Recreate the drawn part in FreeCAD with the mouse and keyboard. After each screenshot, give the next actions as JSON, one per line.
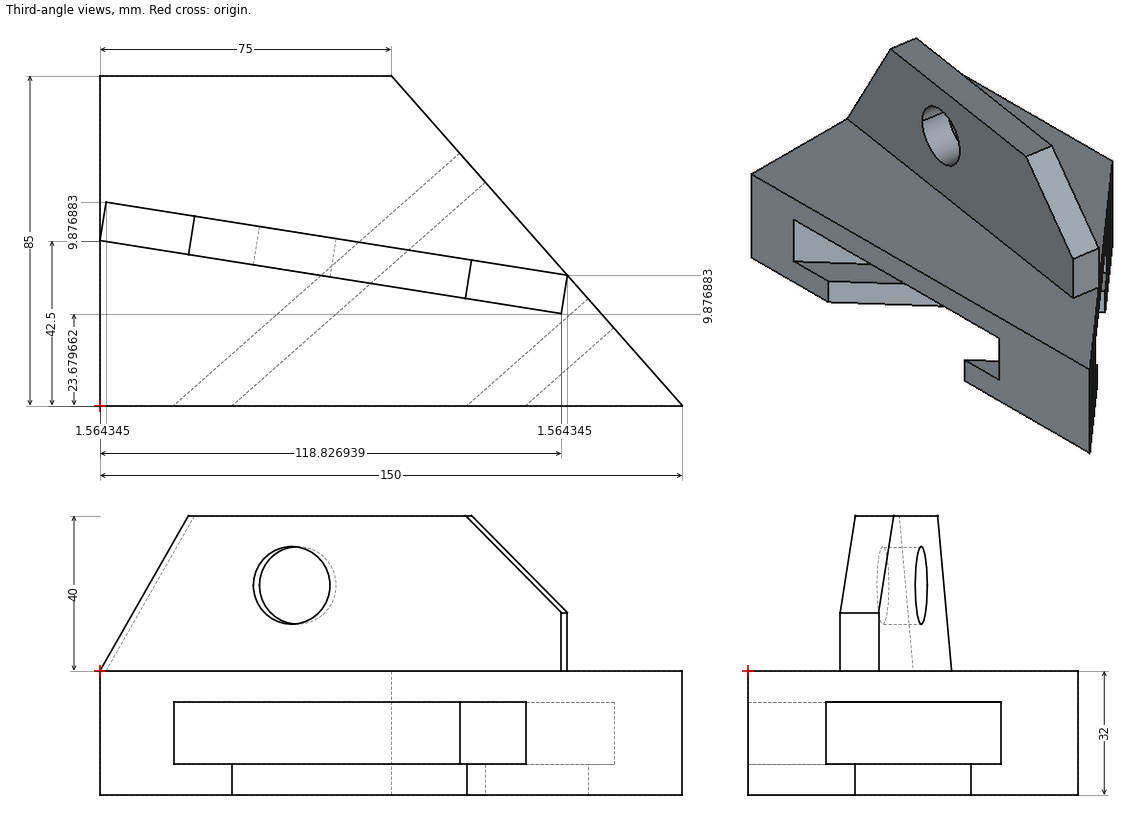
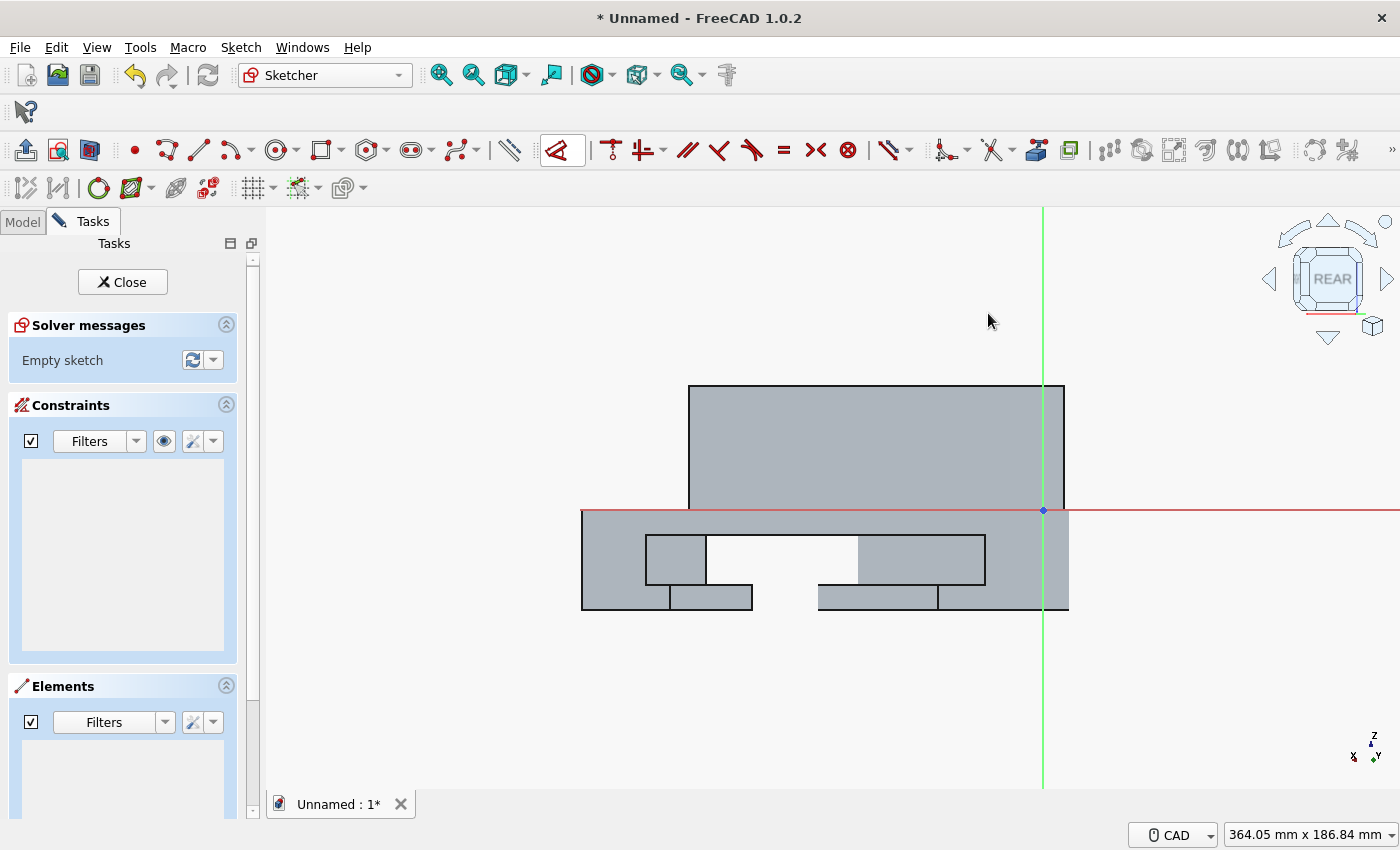
{"action": "key", "text": "g m"}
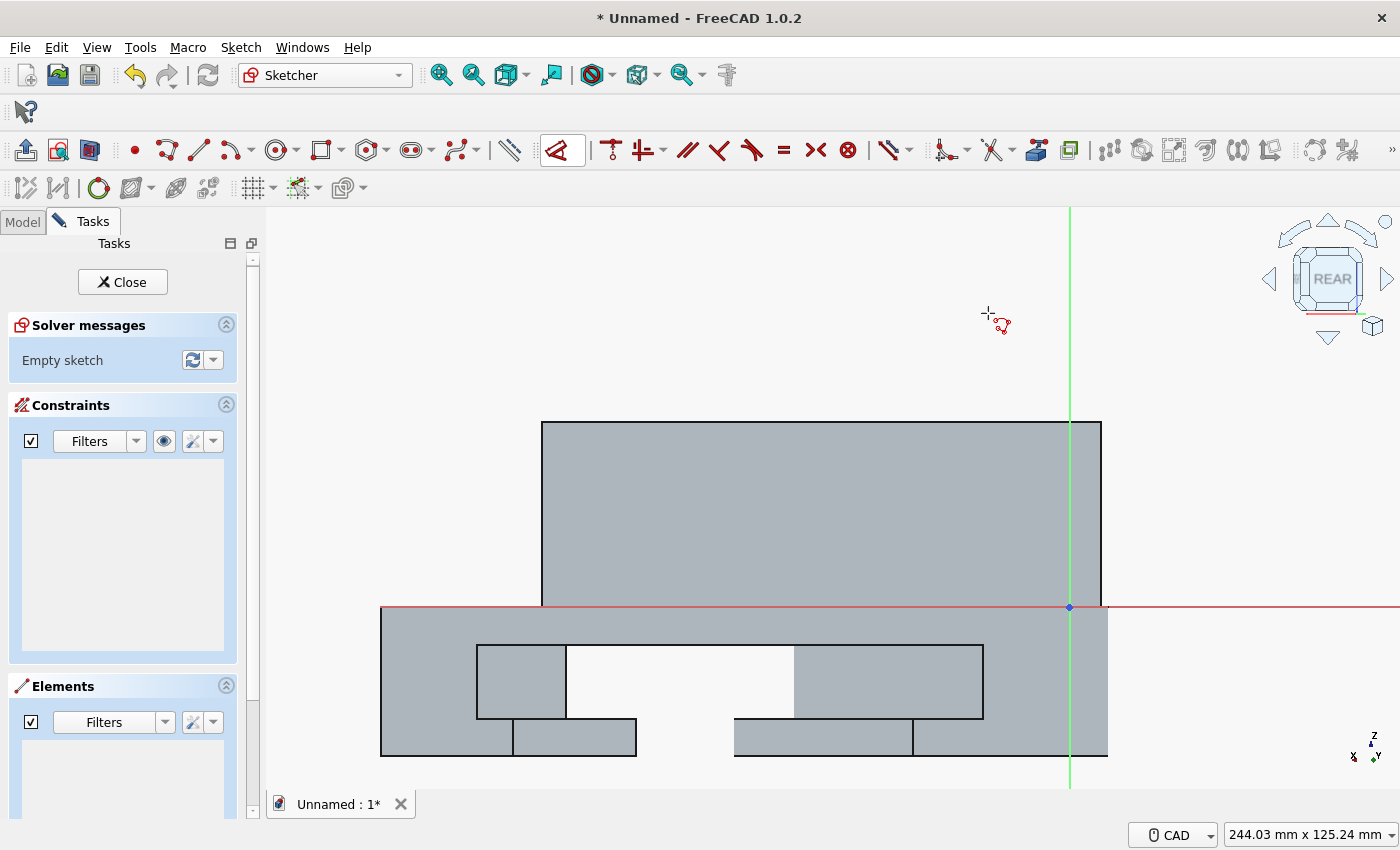
{"action": "left_click", "coordinate": [1101, 607]}
{"action": "left_click", "coordinate": [1101, 392]}
{"action": "left_click", "coordinate": [976, 392]}
{"action": "left_click", "coordinate": [1101, 607]}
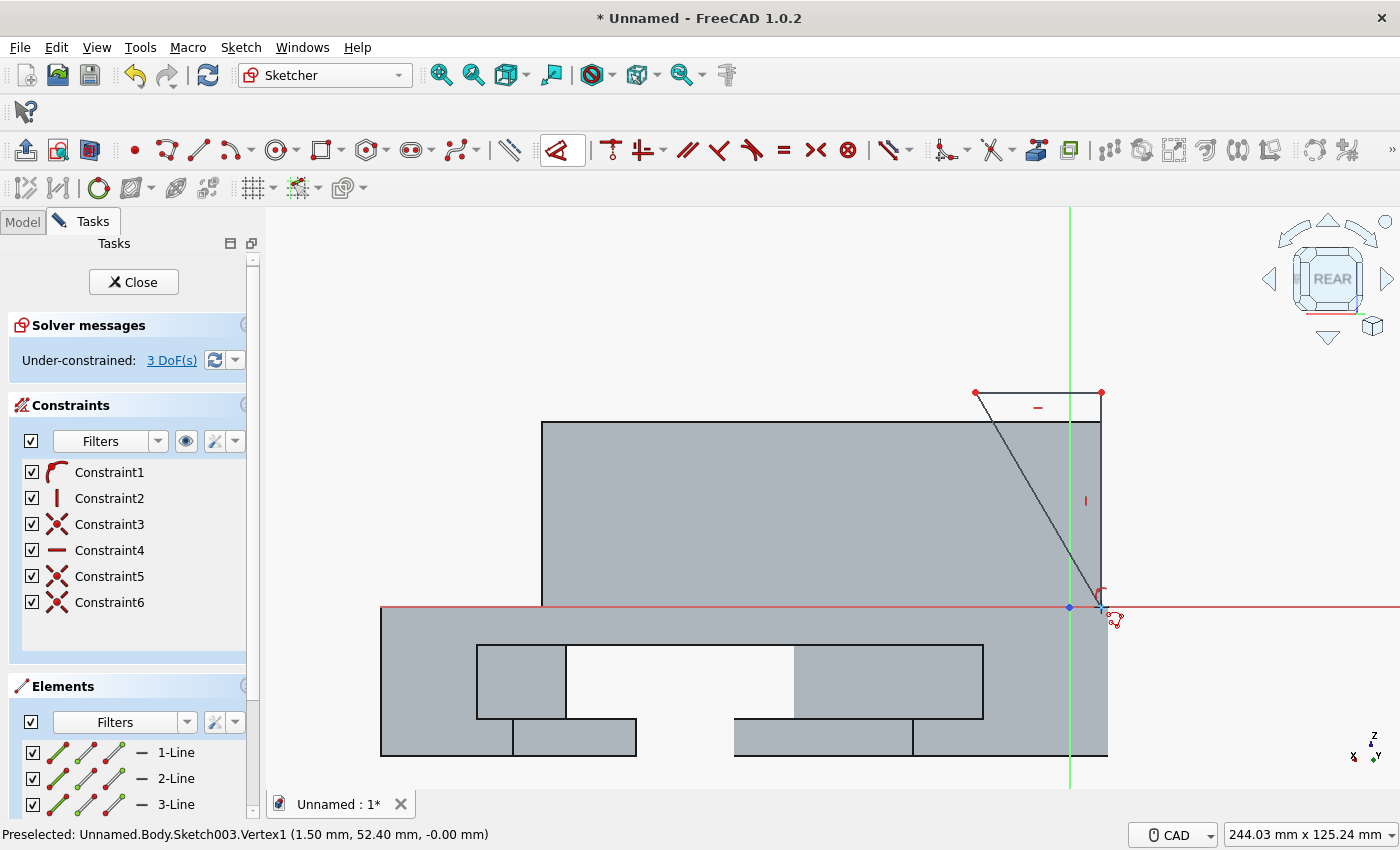
{"action": "left_click", "coordinate": [691, 388]}
{"action": "left_click", "coordinate": [428, 388]}
{"action": "left_click", "coordinate": [542, 538]}
{"action": "left_click", "coordinate": [691, 389]}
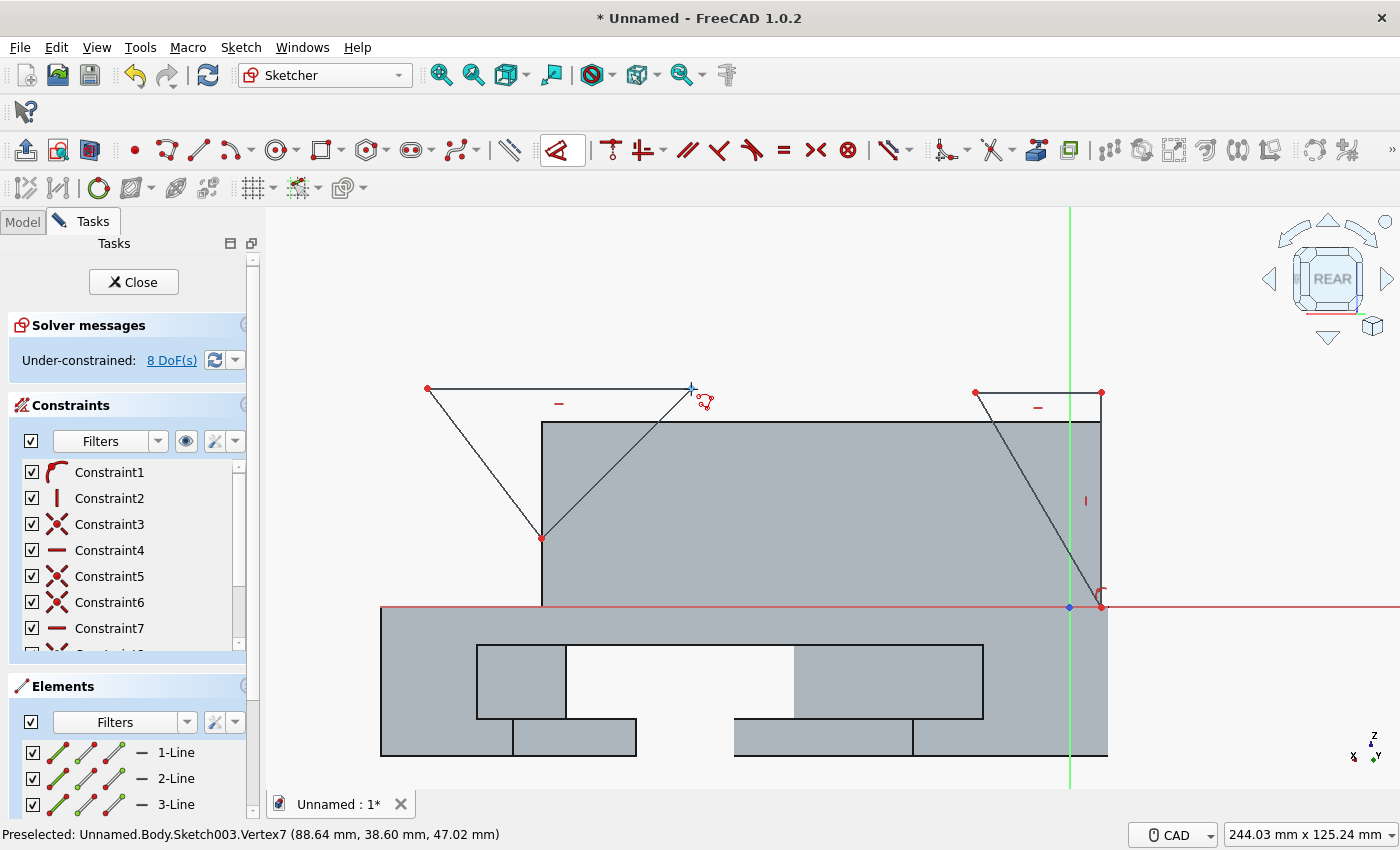
{"action": "key", "text": "g c"}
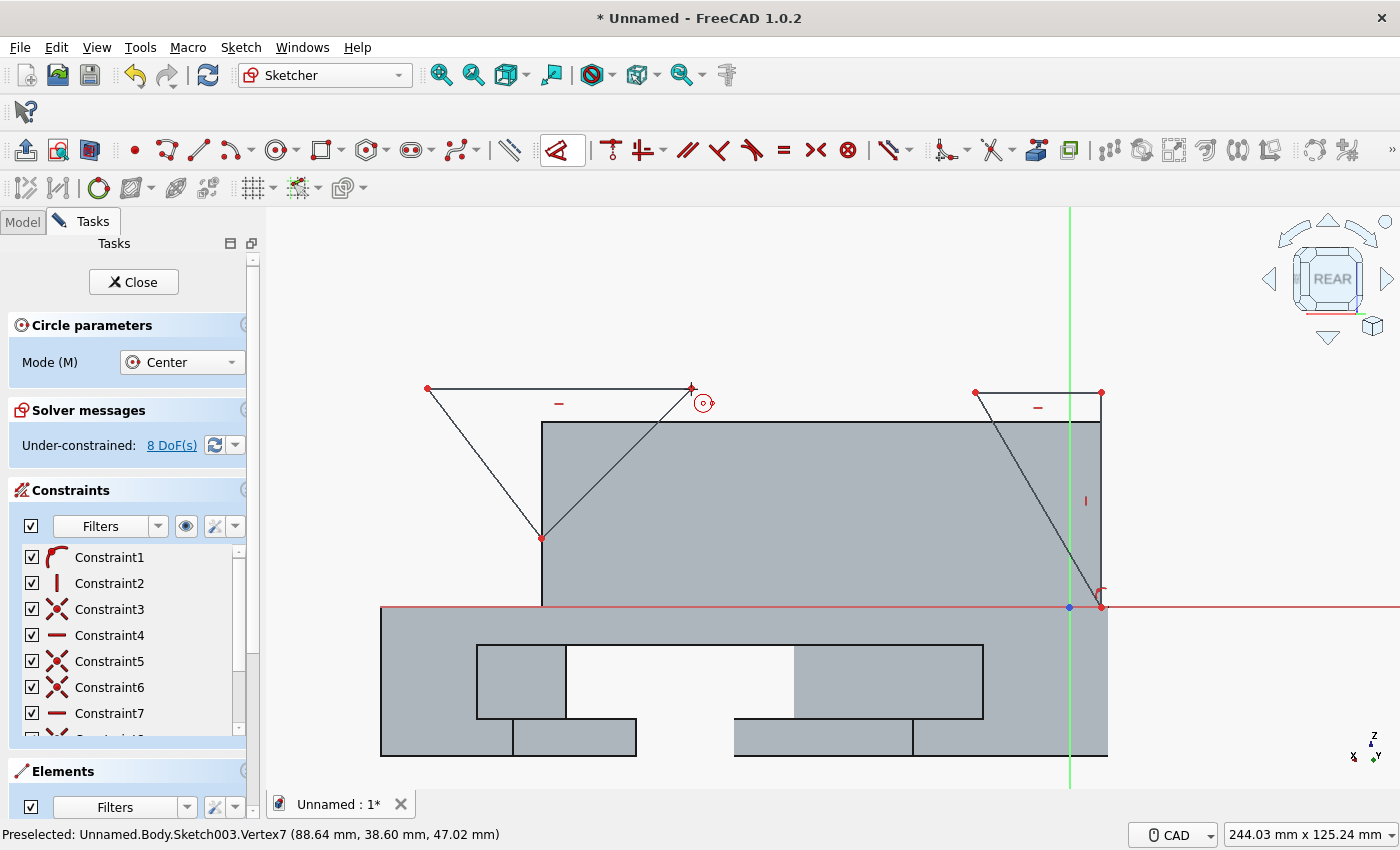
{"action": "left_click", "coordinate": [868, 505]}
{"action": "left_click", "coordinate": [901, 472]}
{"action": "key", "text": "Escape"}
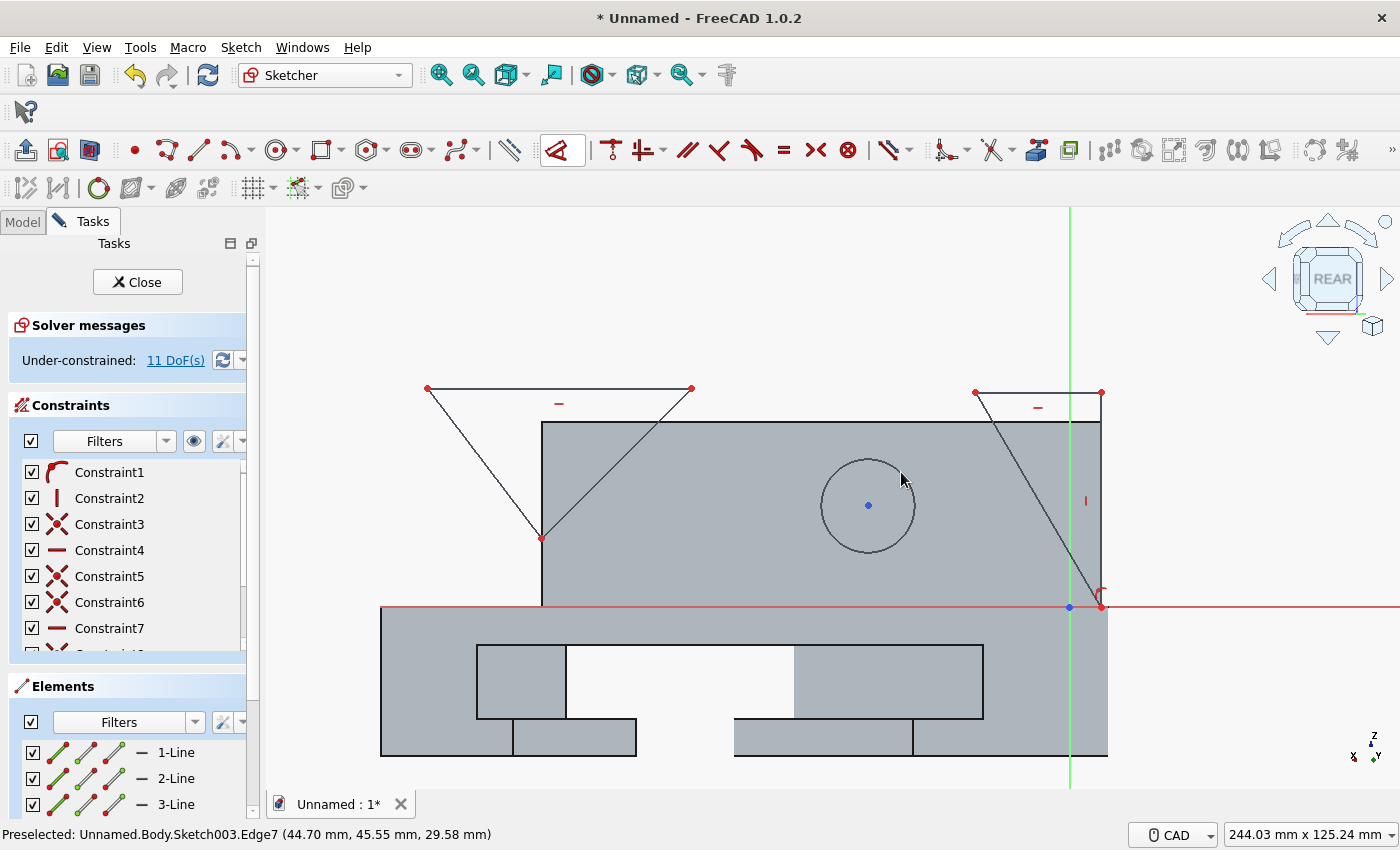
{"action": "left_click", "coordinate": [901, 473]}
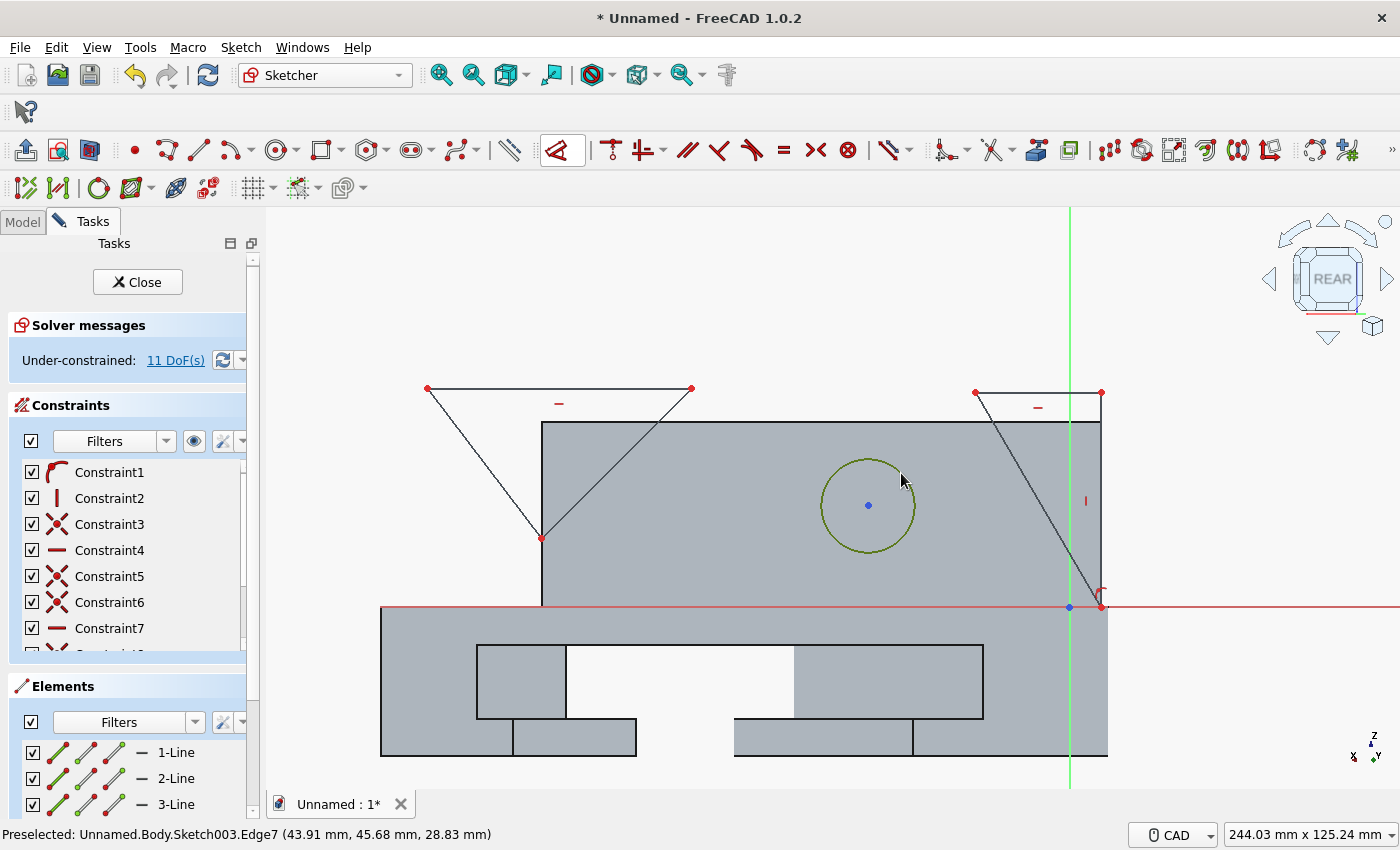
{"action": "key", "text": "k o"}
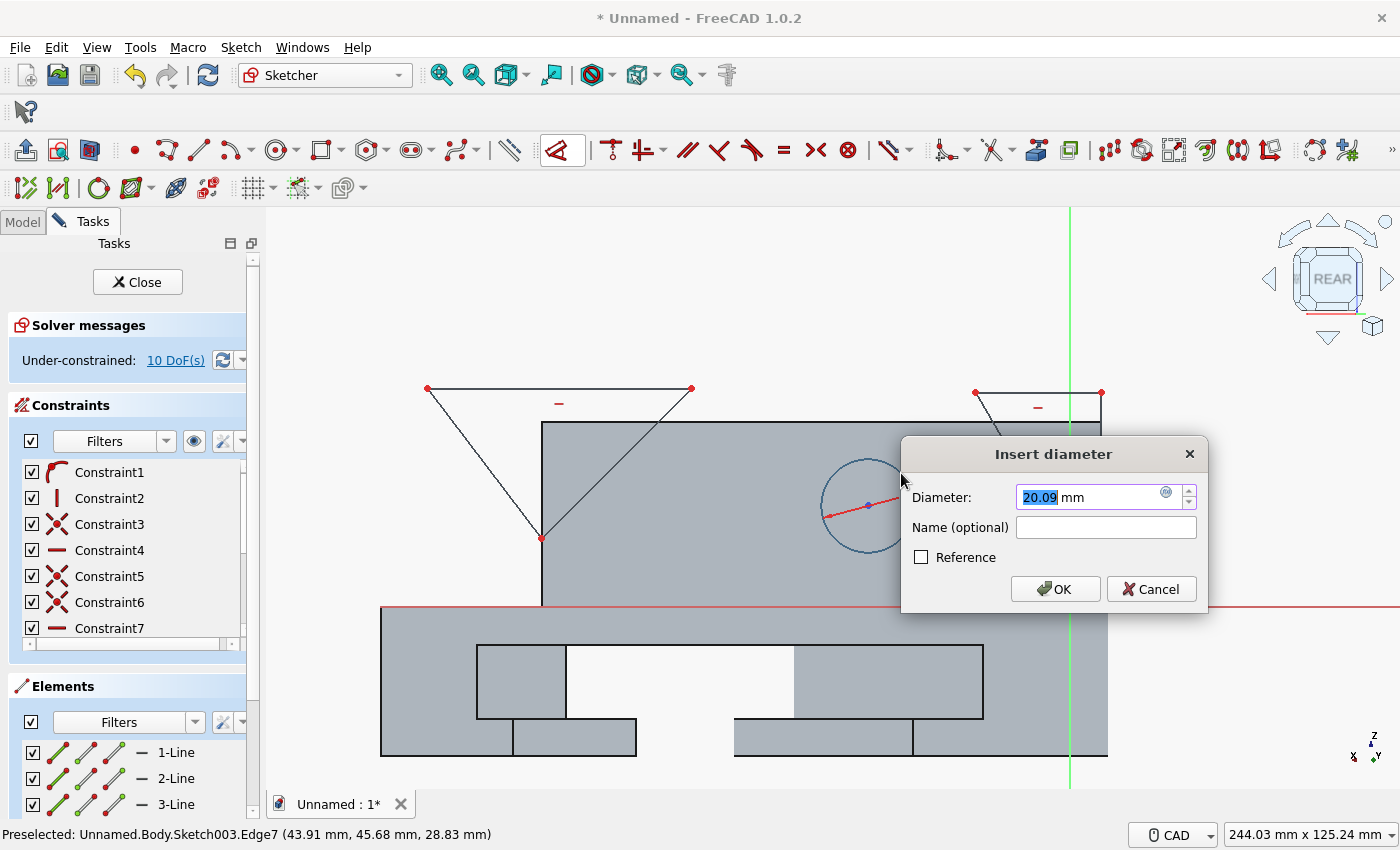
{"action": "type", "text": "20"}
{"action": "key", "text": "Return"}